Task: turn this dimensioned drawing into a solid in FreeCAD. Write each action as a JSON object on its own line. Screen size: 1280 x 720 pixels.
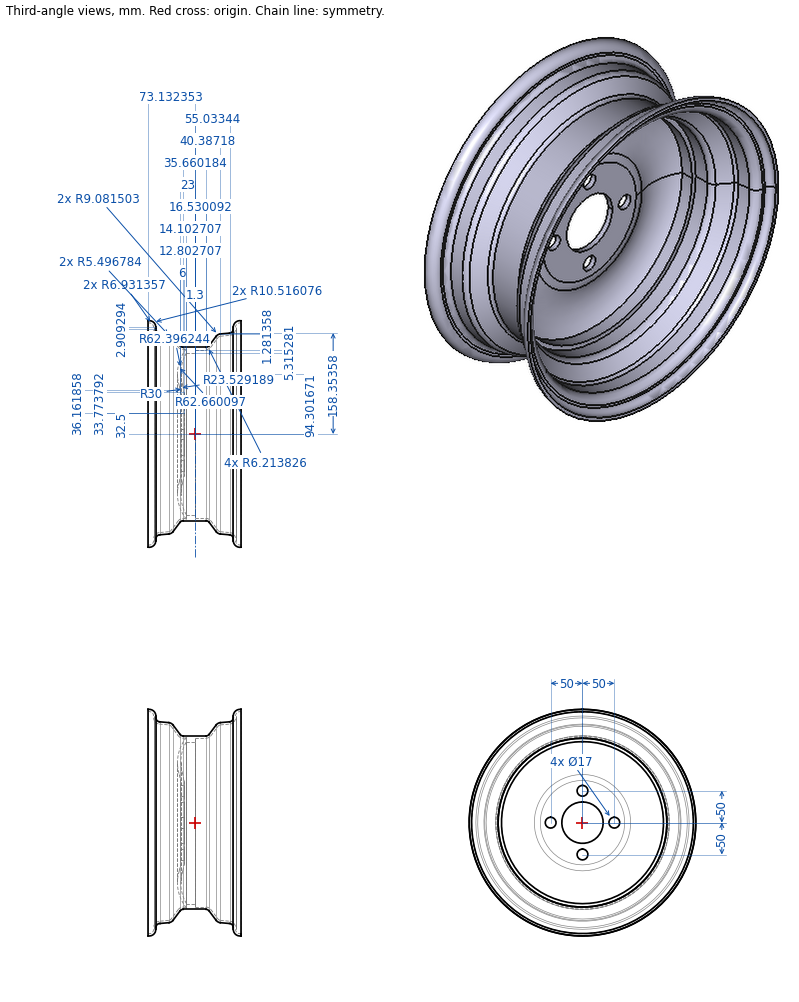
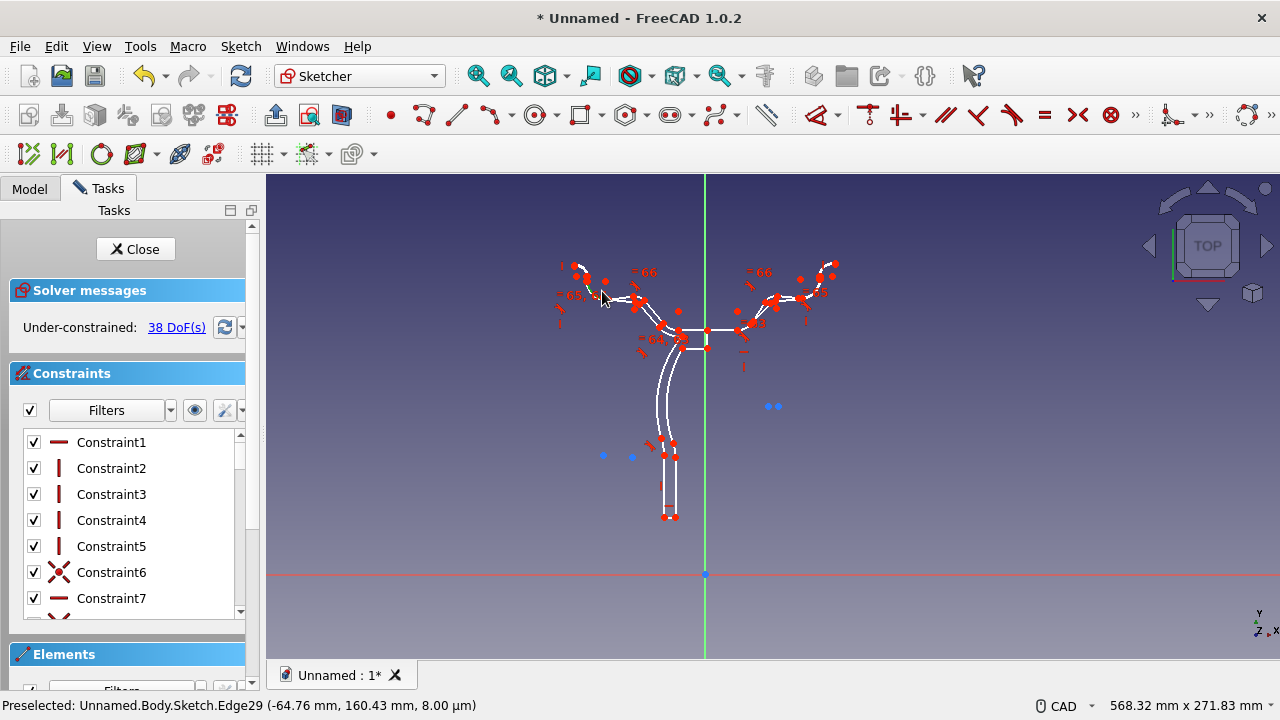
{"action": "scroll", "coordinate": [665, 333], "scroll_direction": "up", "scroll_amount": 5}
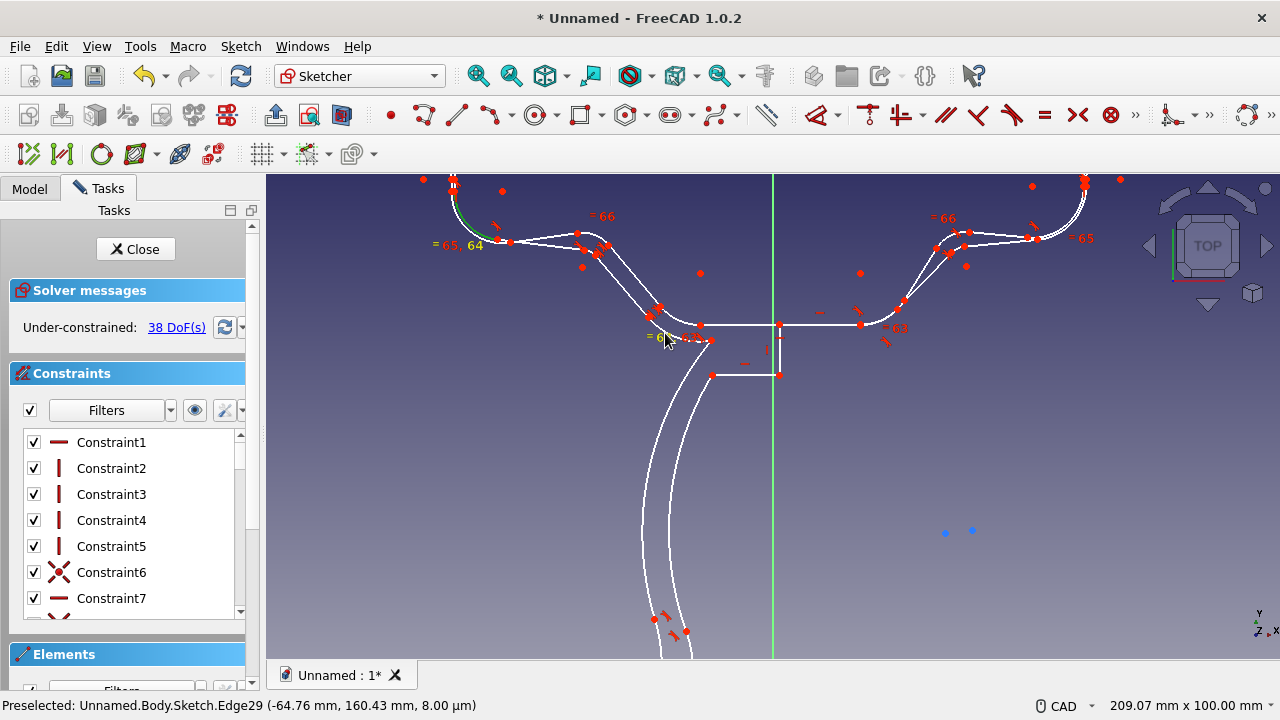
{"action": "left_click", "coordinate": [659, 327]}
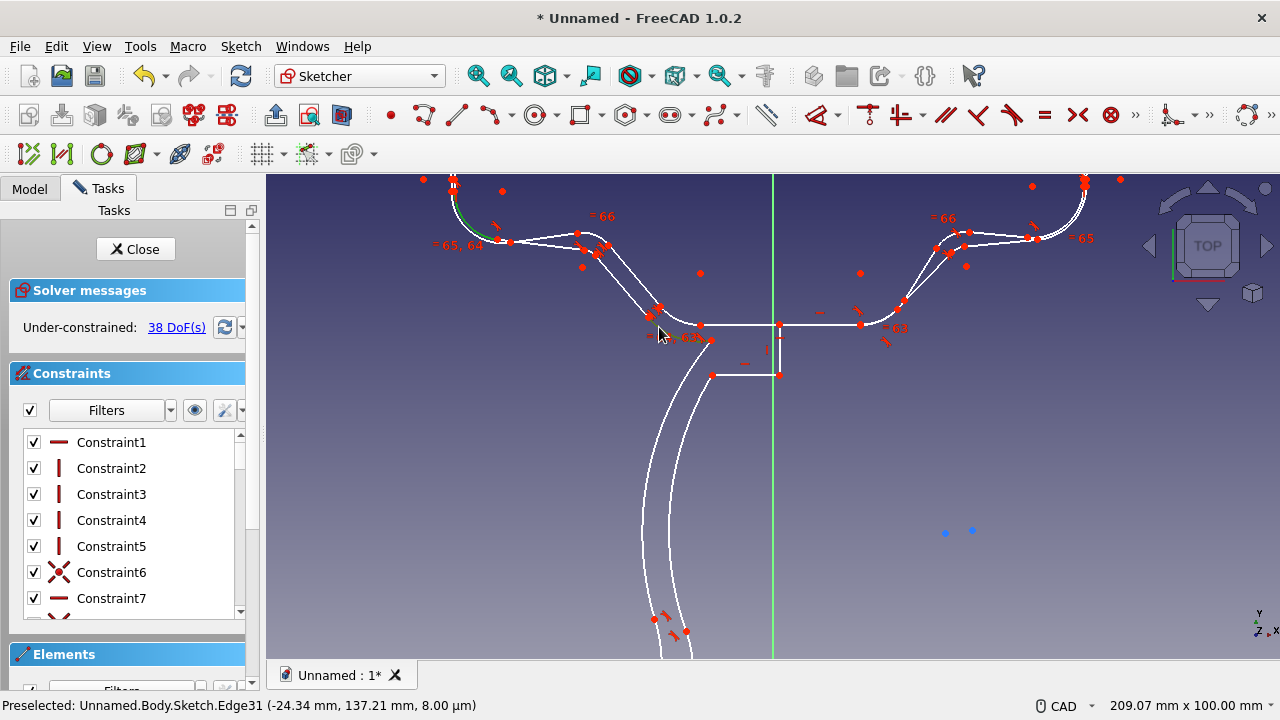
{"action": "scroll", "coordinate": [869, 324], "scroll_direction": "up", "scroll_amount": 9}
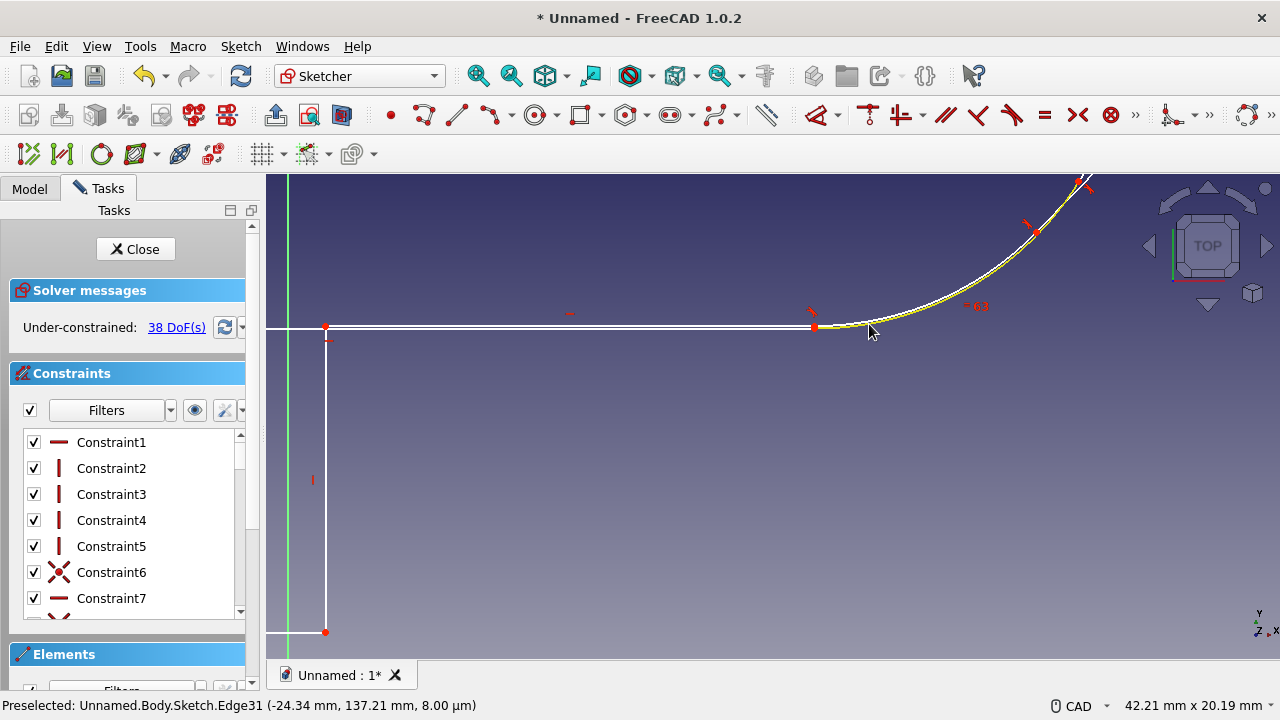
{"action": "scroll", "coordinate": [864, 322], "scroll_direction": "up", "scroll_amount": 4}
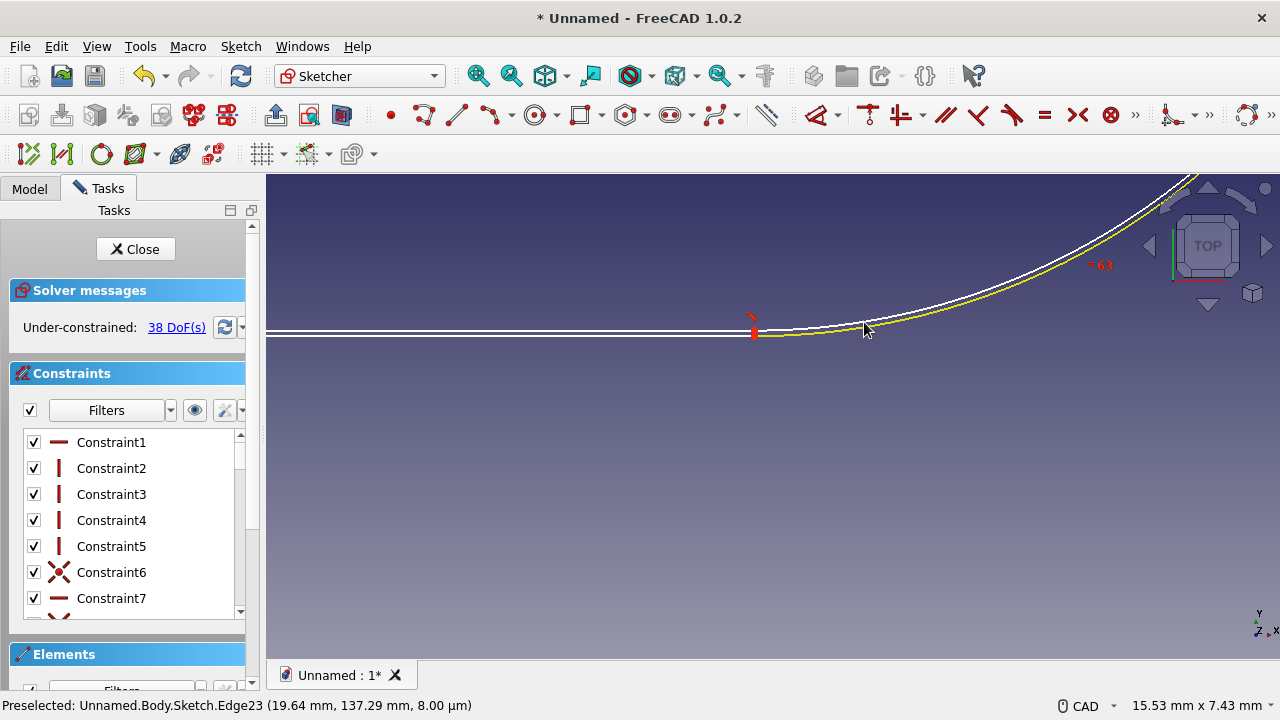
{"action": "left_click", "coordinate": [1021, 276]}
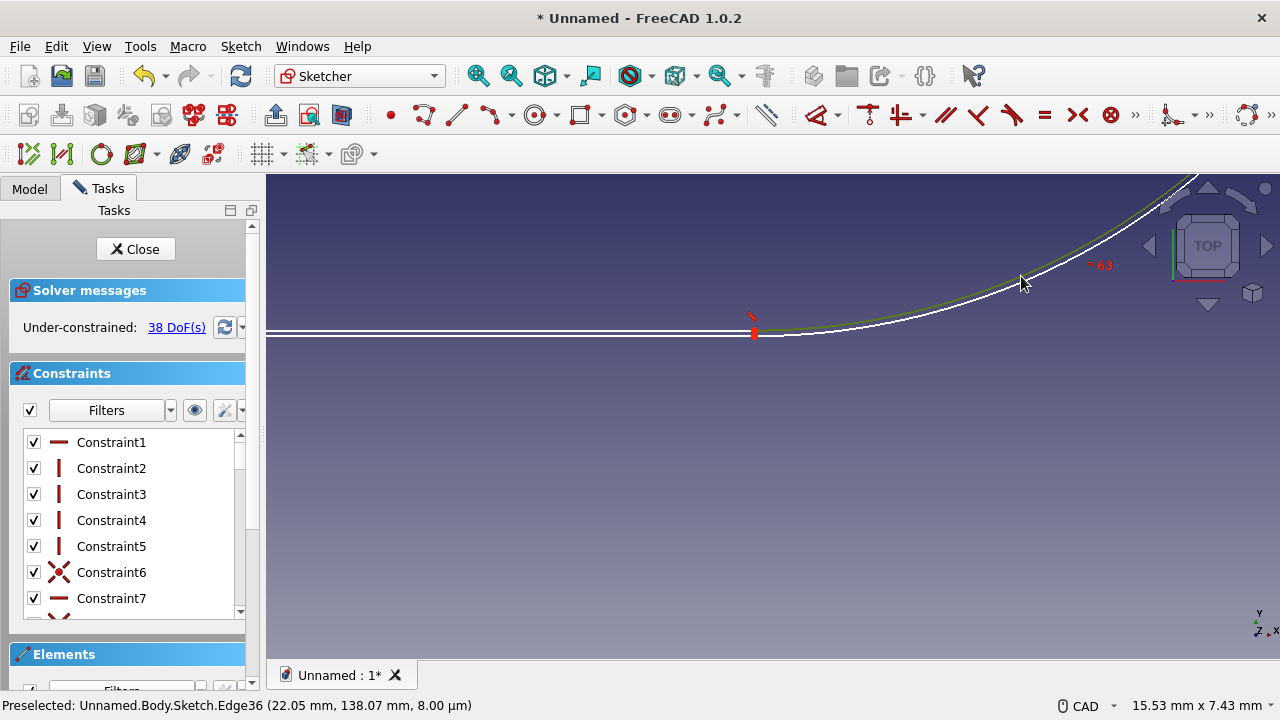
{"action": "scroll", "coordinate": [736, 330], "scroll_direction": "down", "scroll_amount": 18}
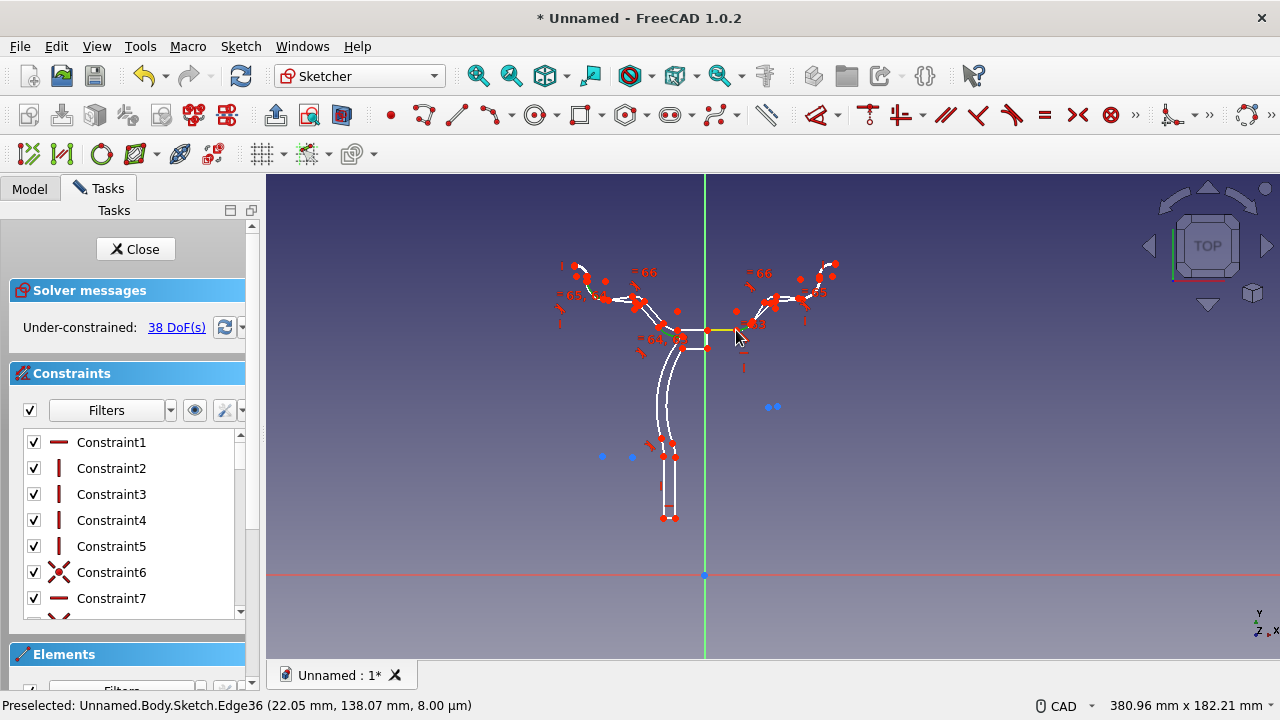
{"action": "scroll", "coordinate": [810, 296], "scroll_direction": "up", "scroll_amount": 14}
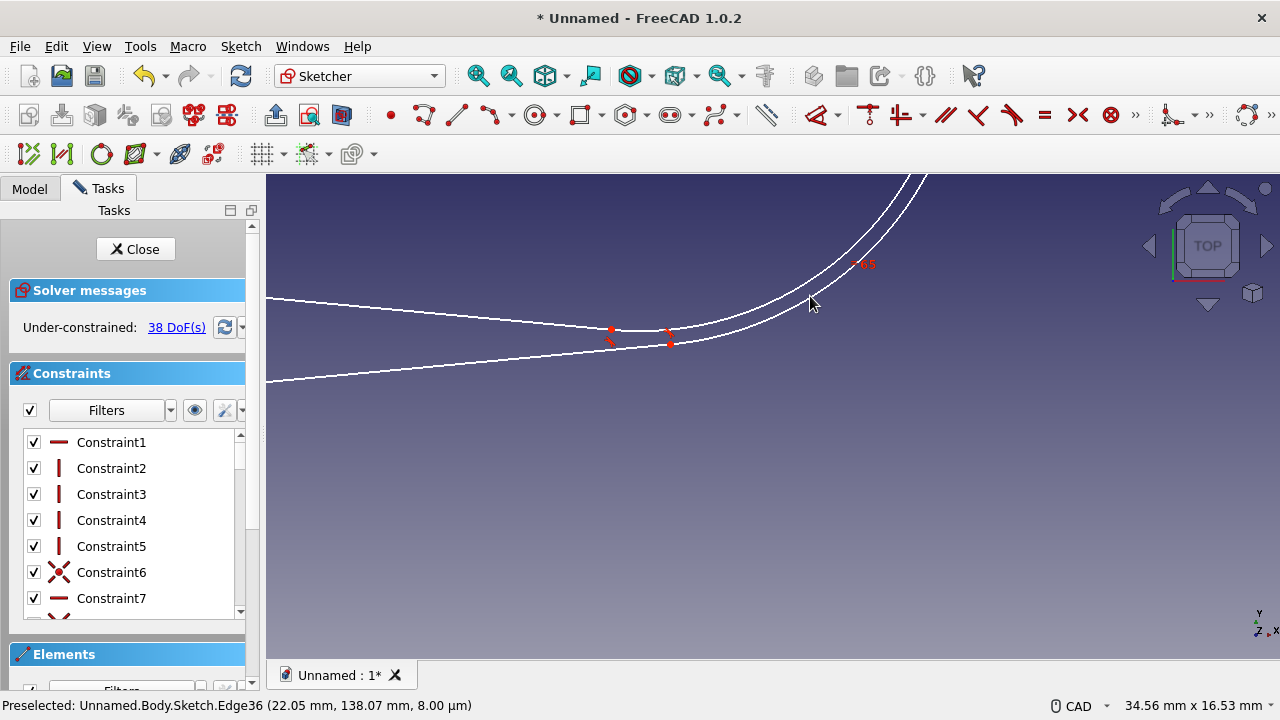
{"action": "left_click", "coordinate": [806, 300]}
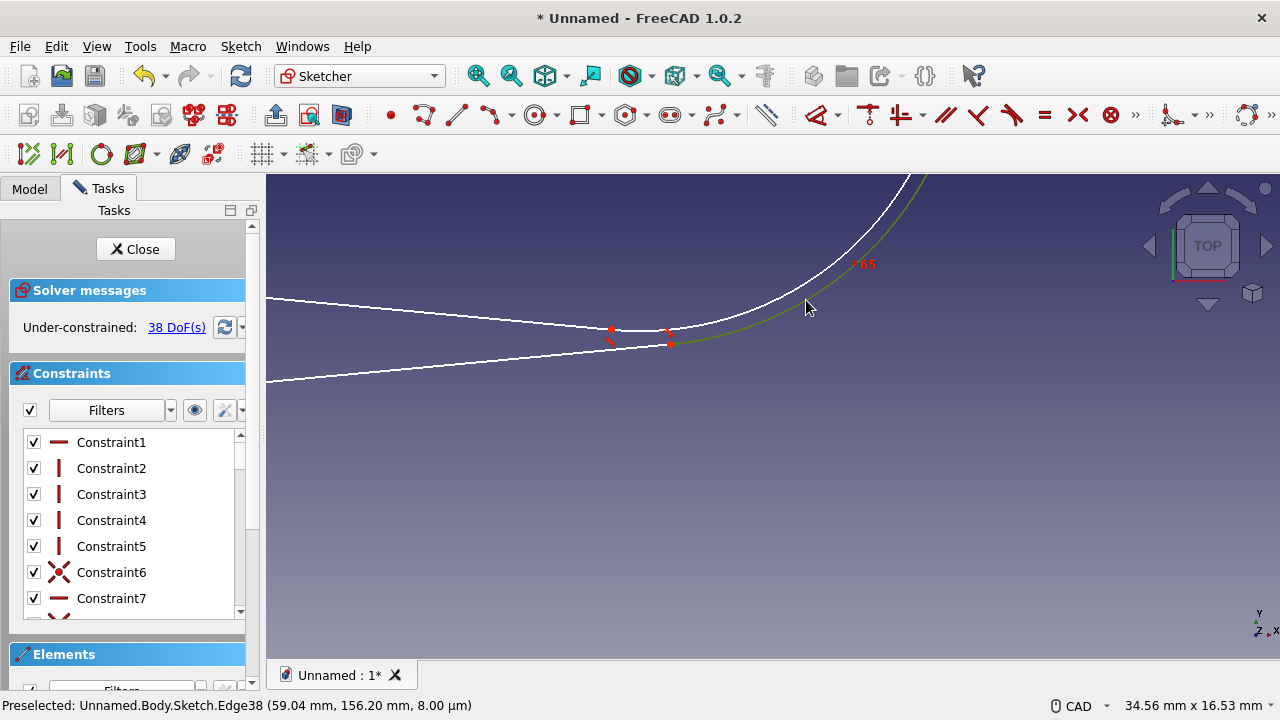
{"action": "key", "text": "e"}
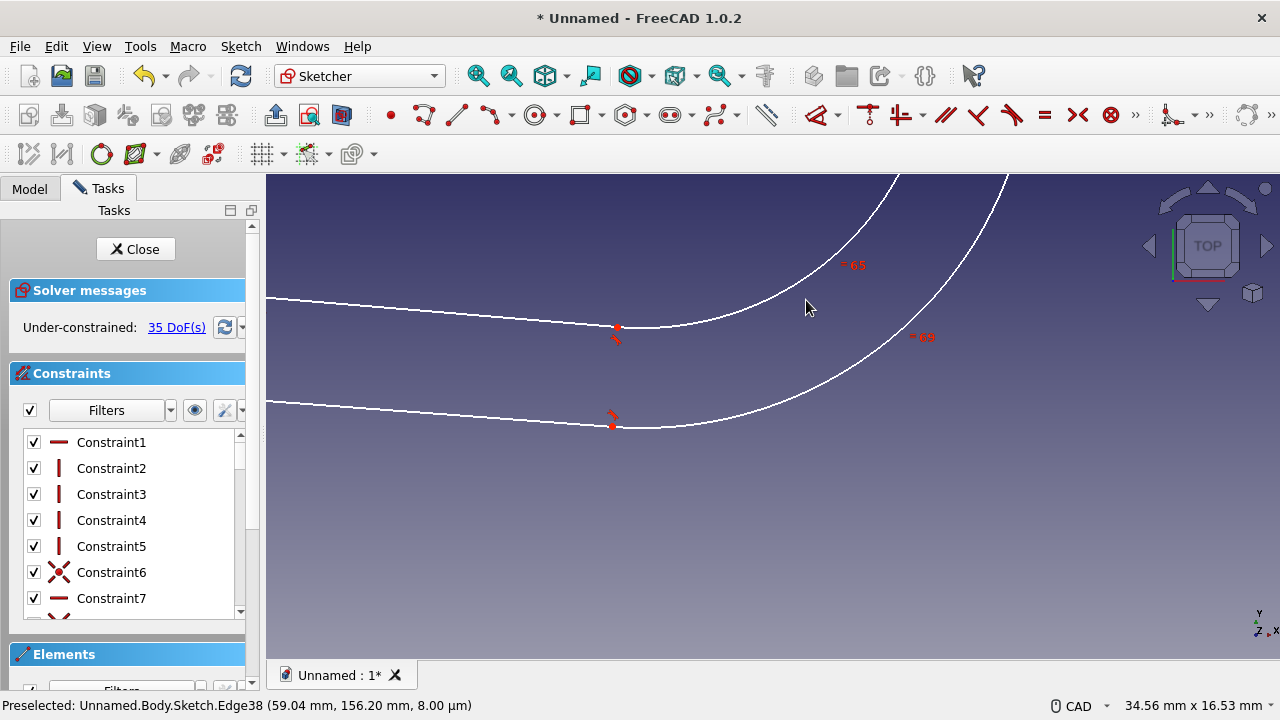
{"action": "scroll", "coordinate": [810, 296], "scroll_direction": "down", "scroll_amount": 14}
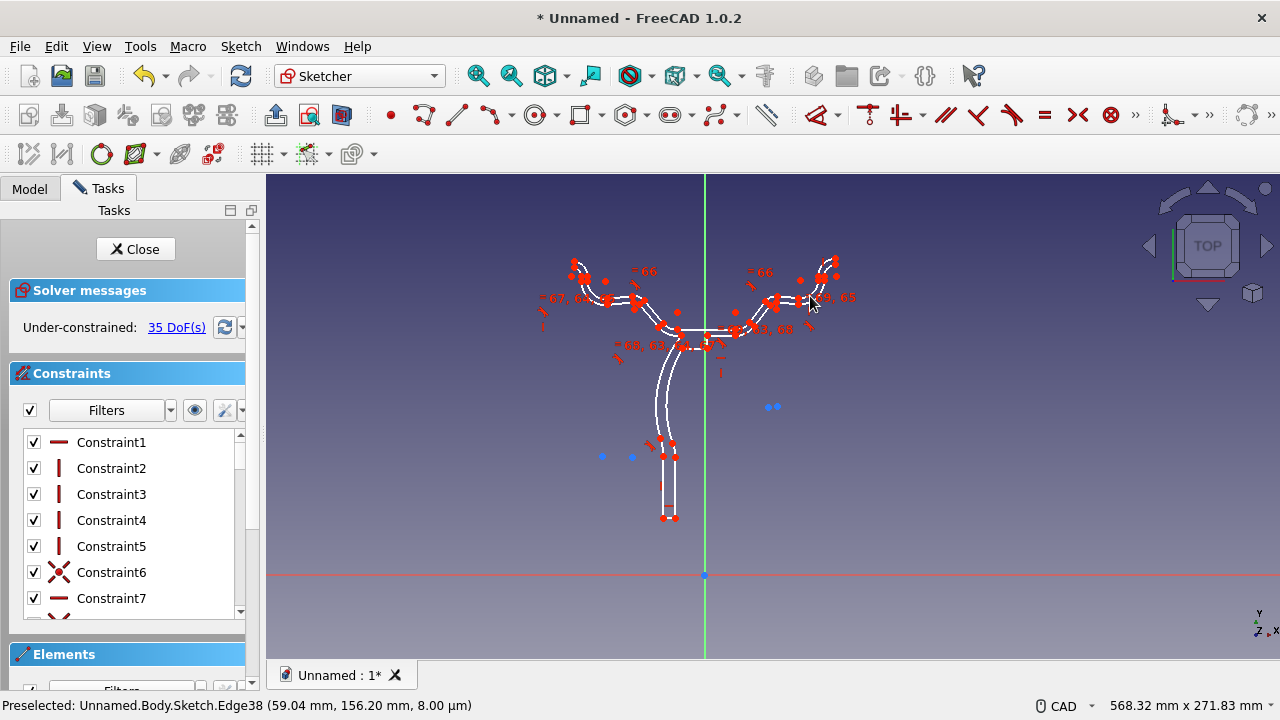
{"action": "scroll", "coordinate": [638, 303], "scroll_direction": "up", "scroll_amount": 10}